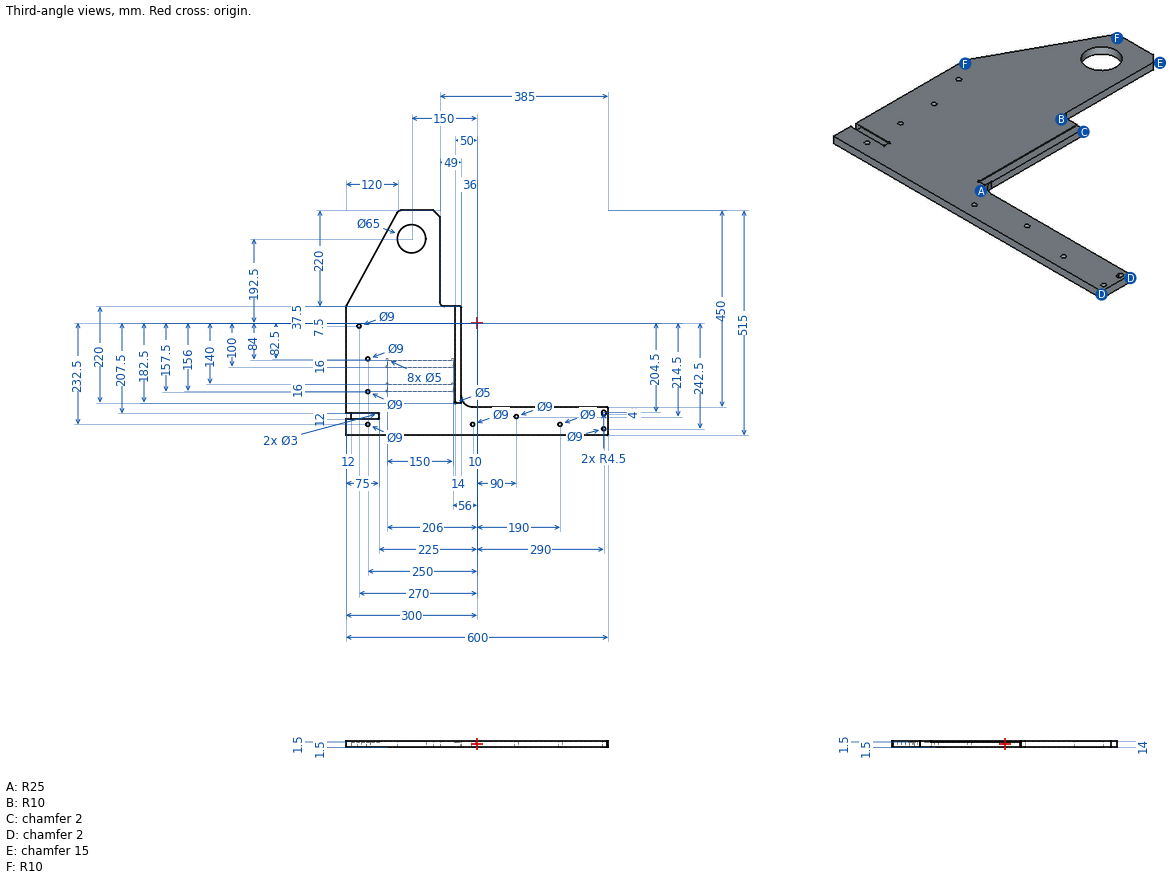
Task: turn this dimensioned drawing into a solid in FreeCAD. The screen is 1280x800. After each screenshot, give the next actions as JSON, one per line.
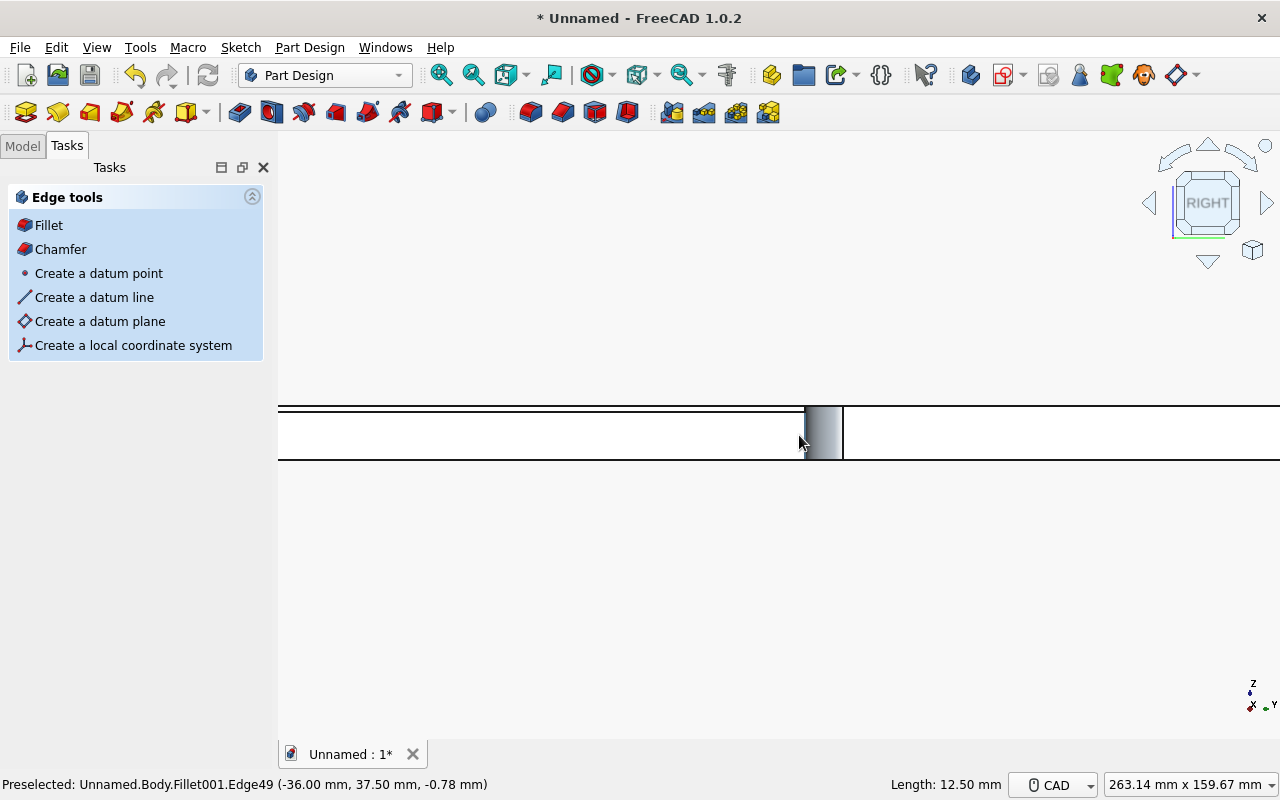
{"action": "left_click", "coordinate": [564, 112]}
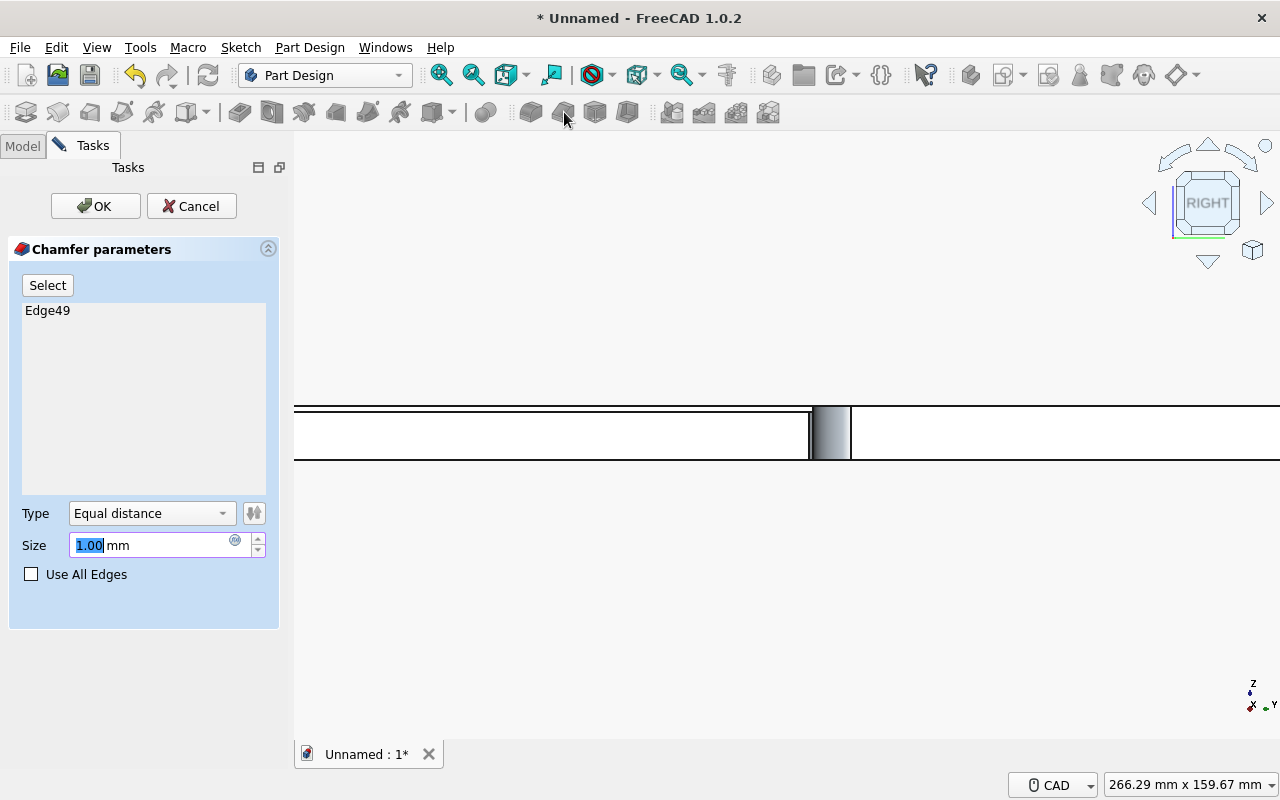
{"action": "type", "text": "2"}
{"action": "key", "text": "Tab"}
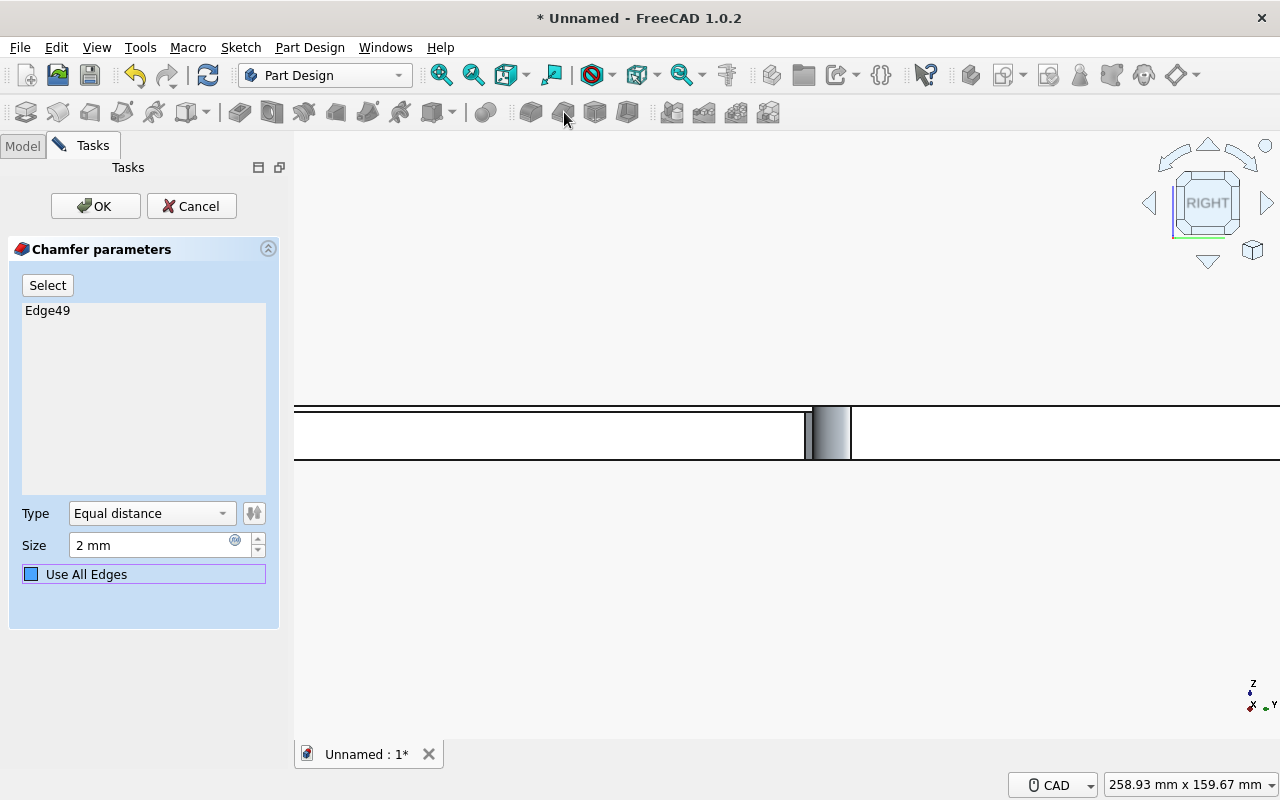
{"action": "left_click", "coordinate": [96, 206]}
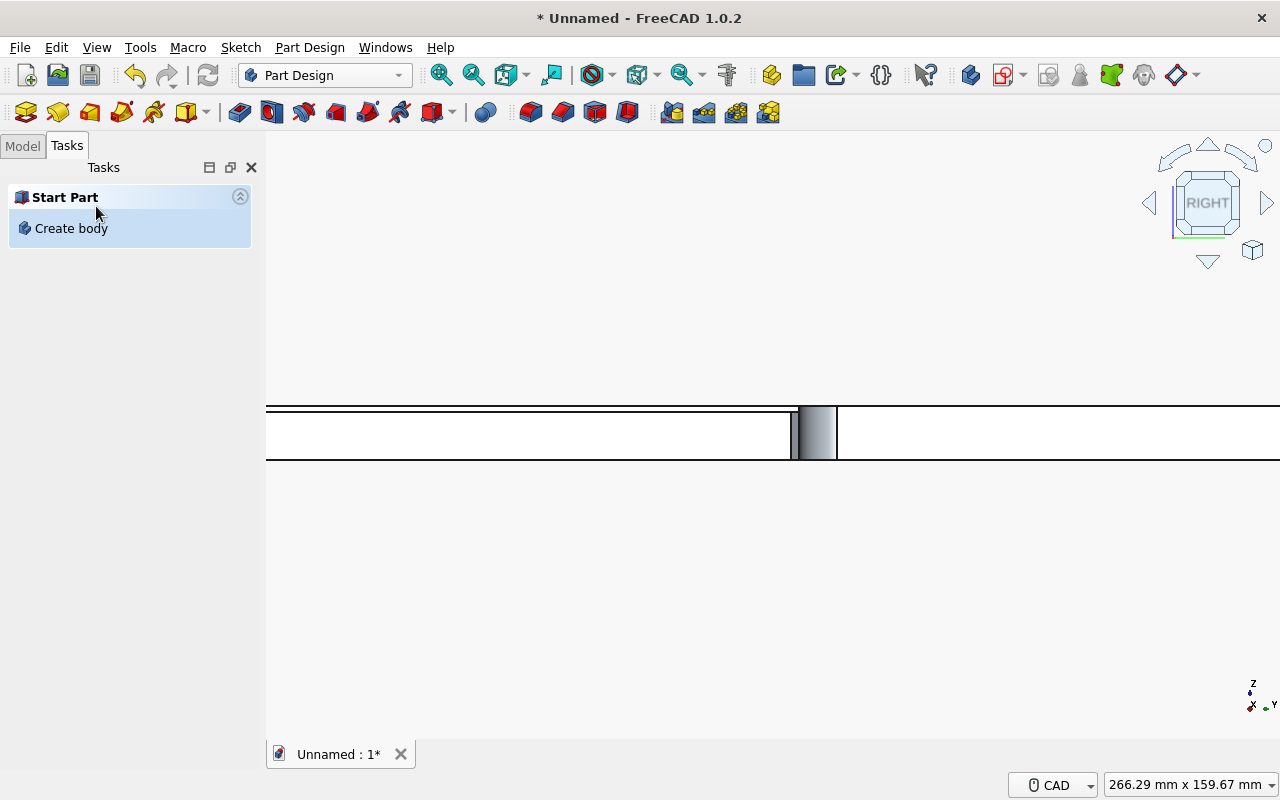
{"action": "left_click", "coordinate": [442, 76]}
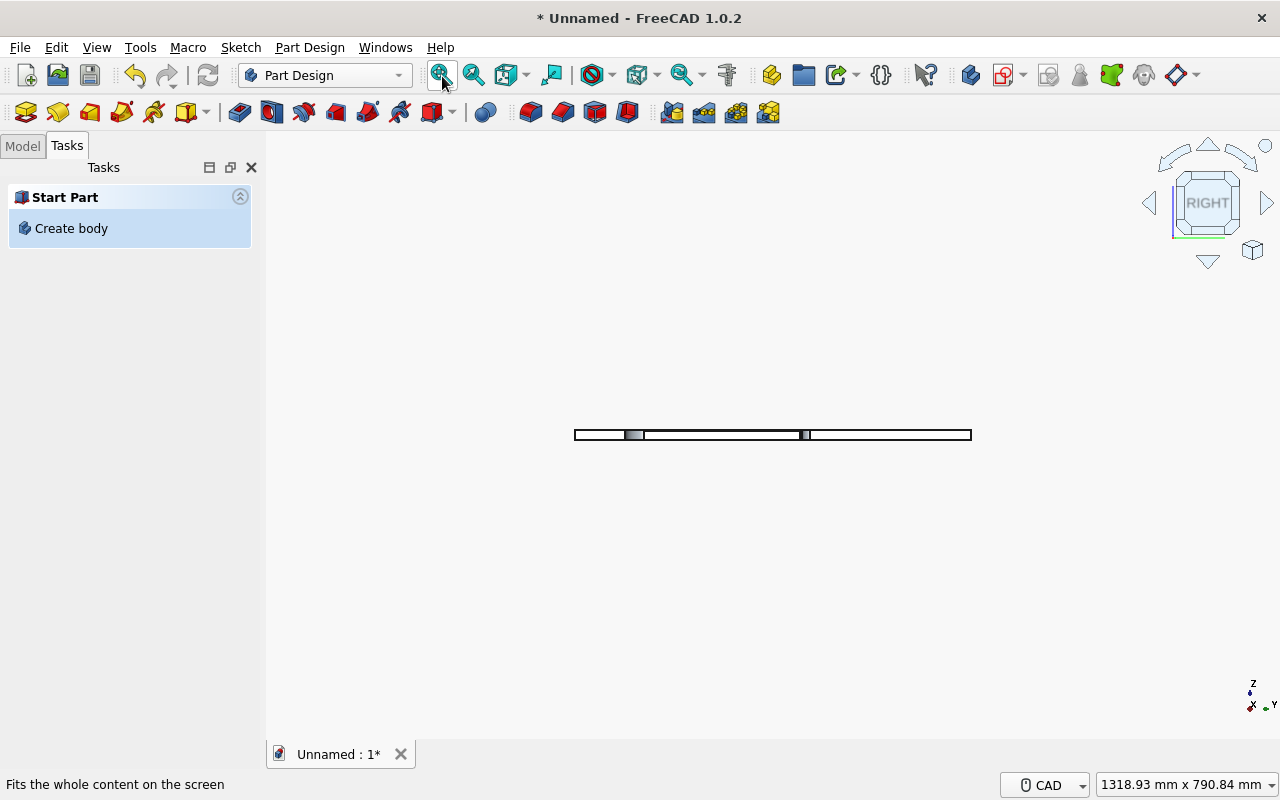
{"action": "scroll", "coordinate": [625, 434], "scroll_direction": "up", "scroll_amount": 7}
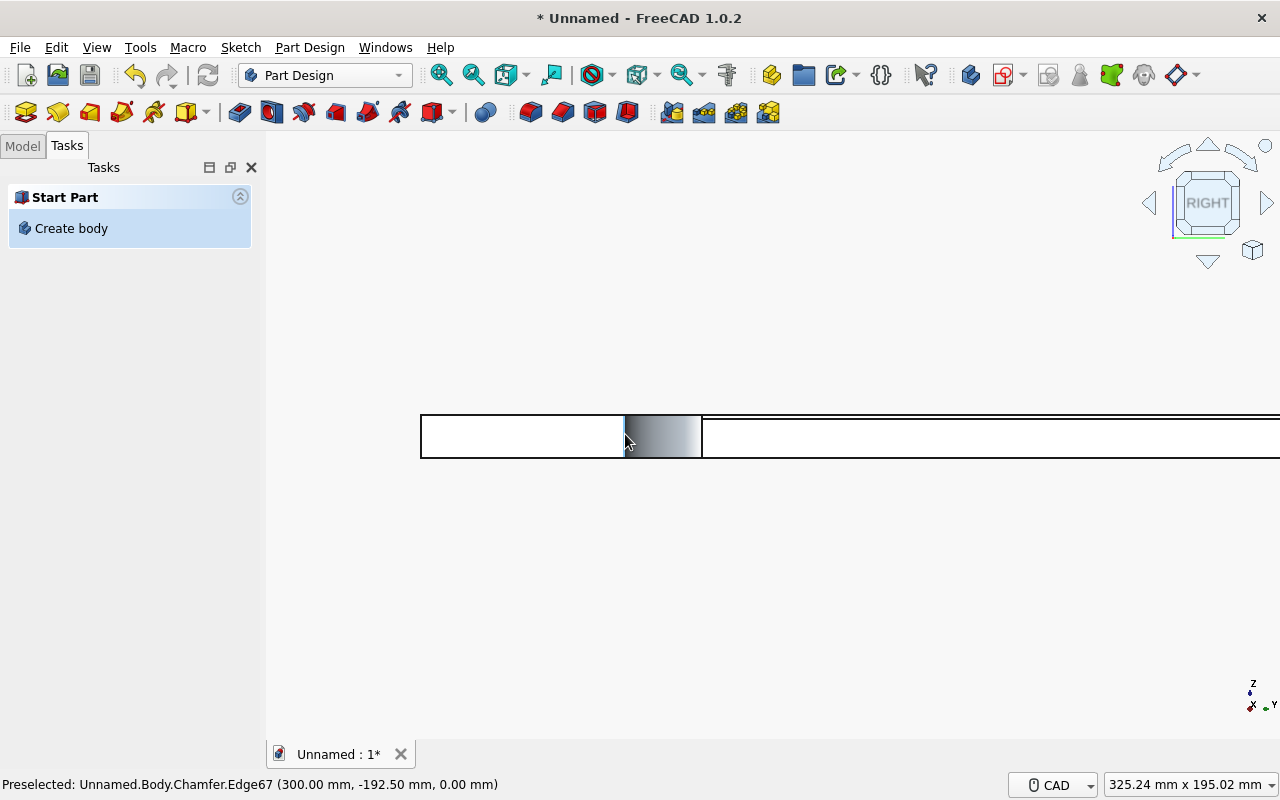
{"action": "left_click", "coordinate": [624, 436]}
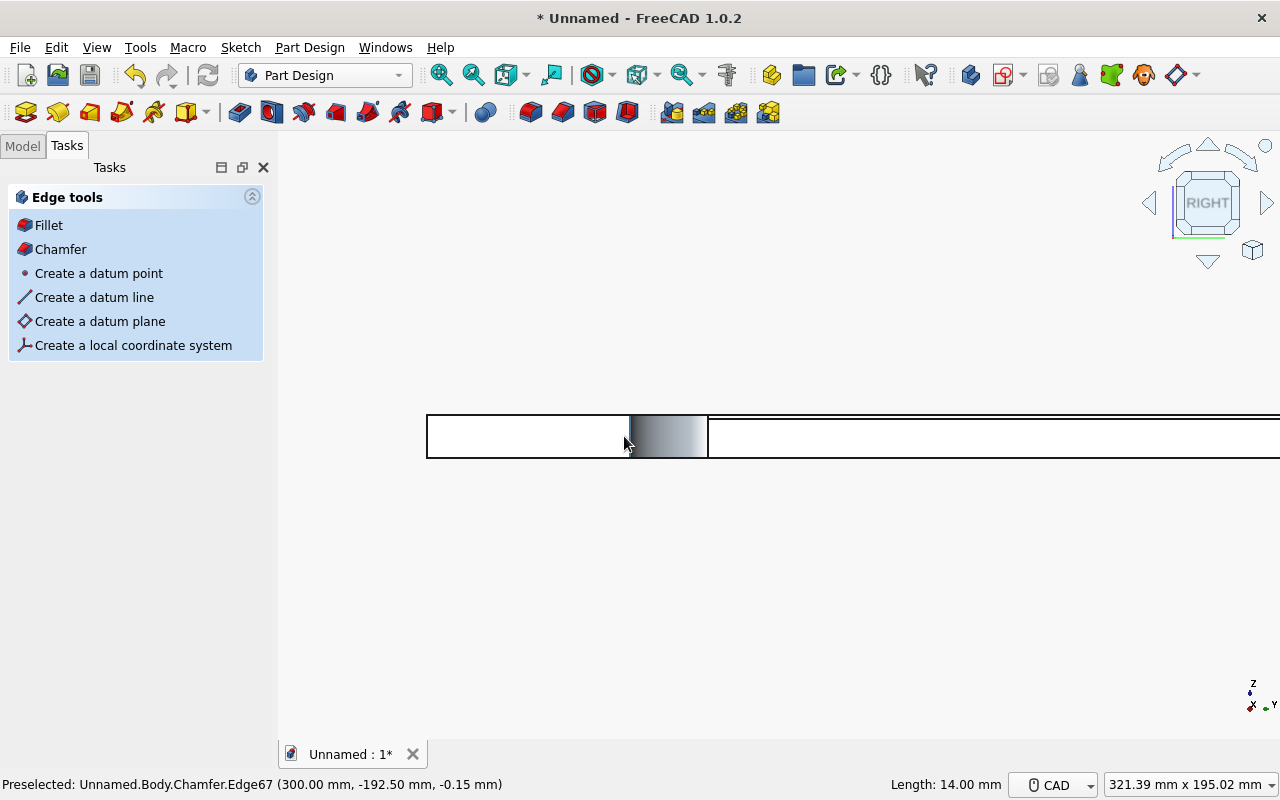
{"action": "left_click", "coordinate": [427, 436], "text": "ctrl"}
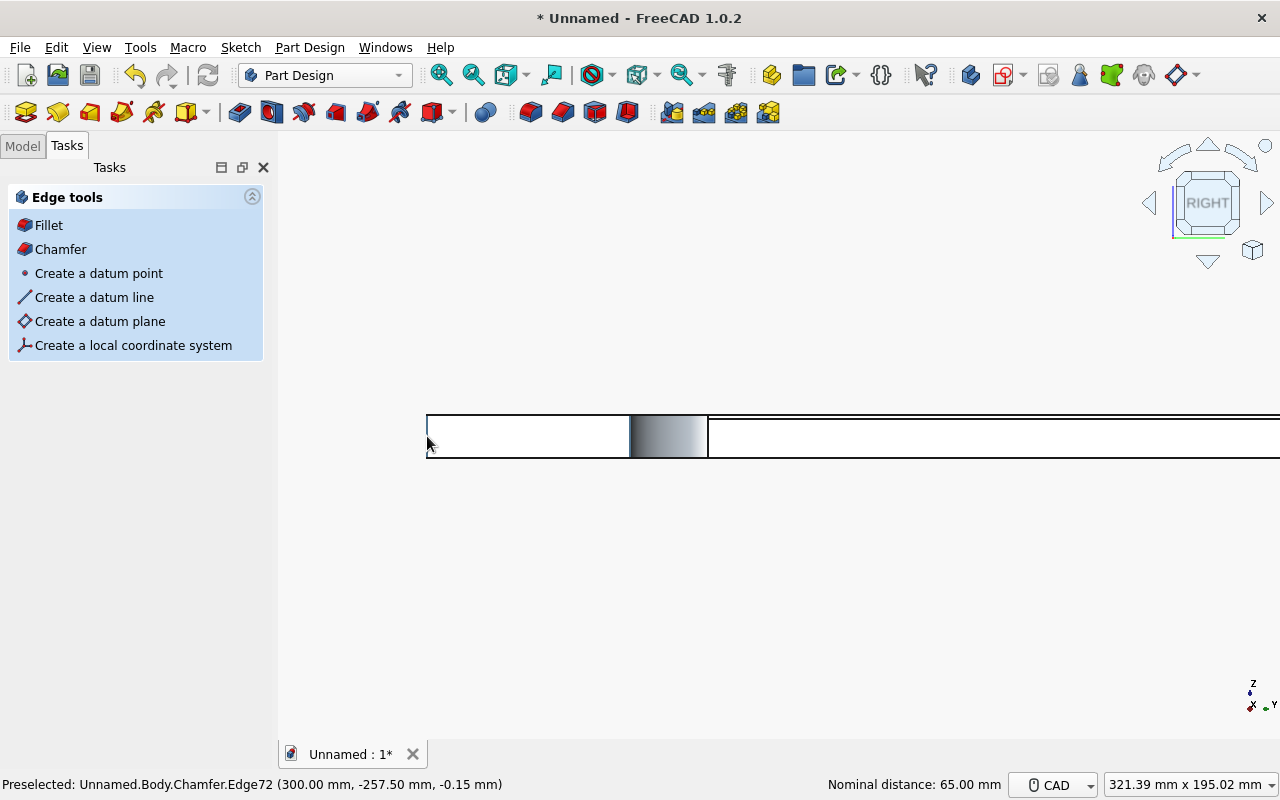
{"action": "left_click", "coordinate": [564, 112]}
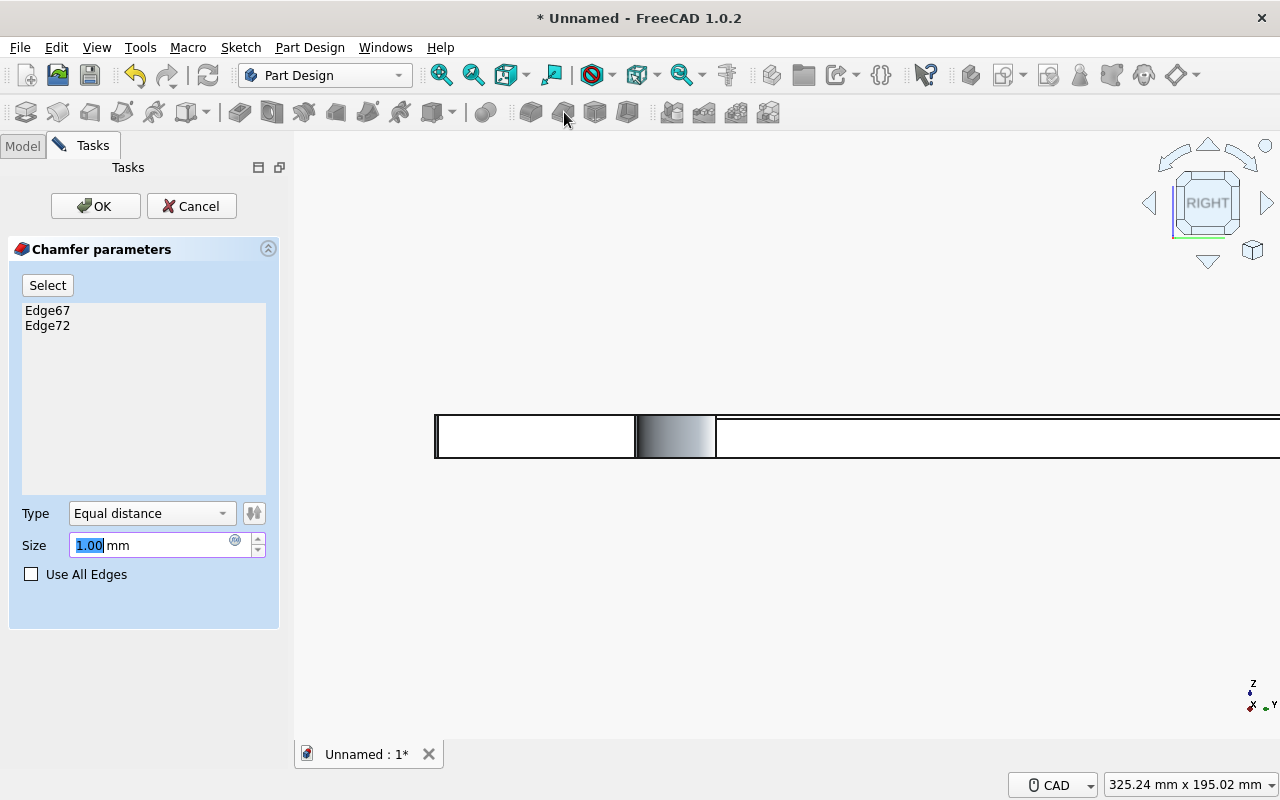
{"action": "type", "text": "2"}
{"action": "key", "text": "Tab"}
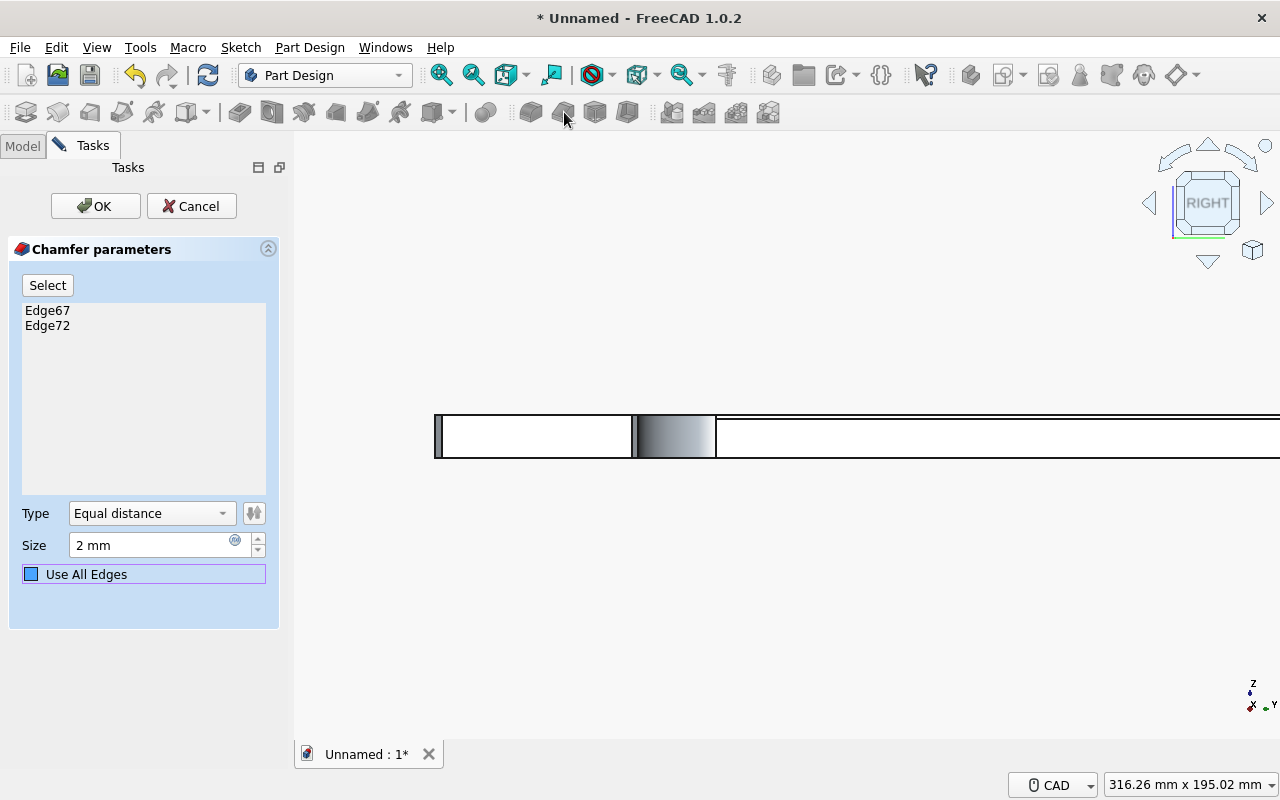
{"action": "left_click", "coordinate": [96, 206]}